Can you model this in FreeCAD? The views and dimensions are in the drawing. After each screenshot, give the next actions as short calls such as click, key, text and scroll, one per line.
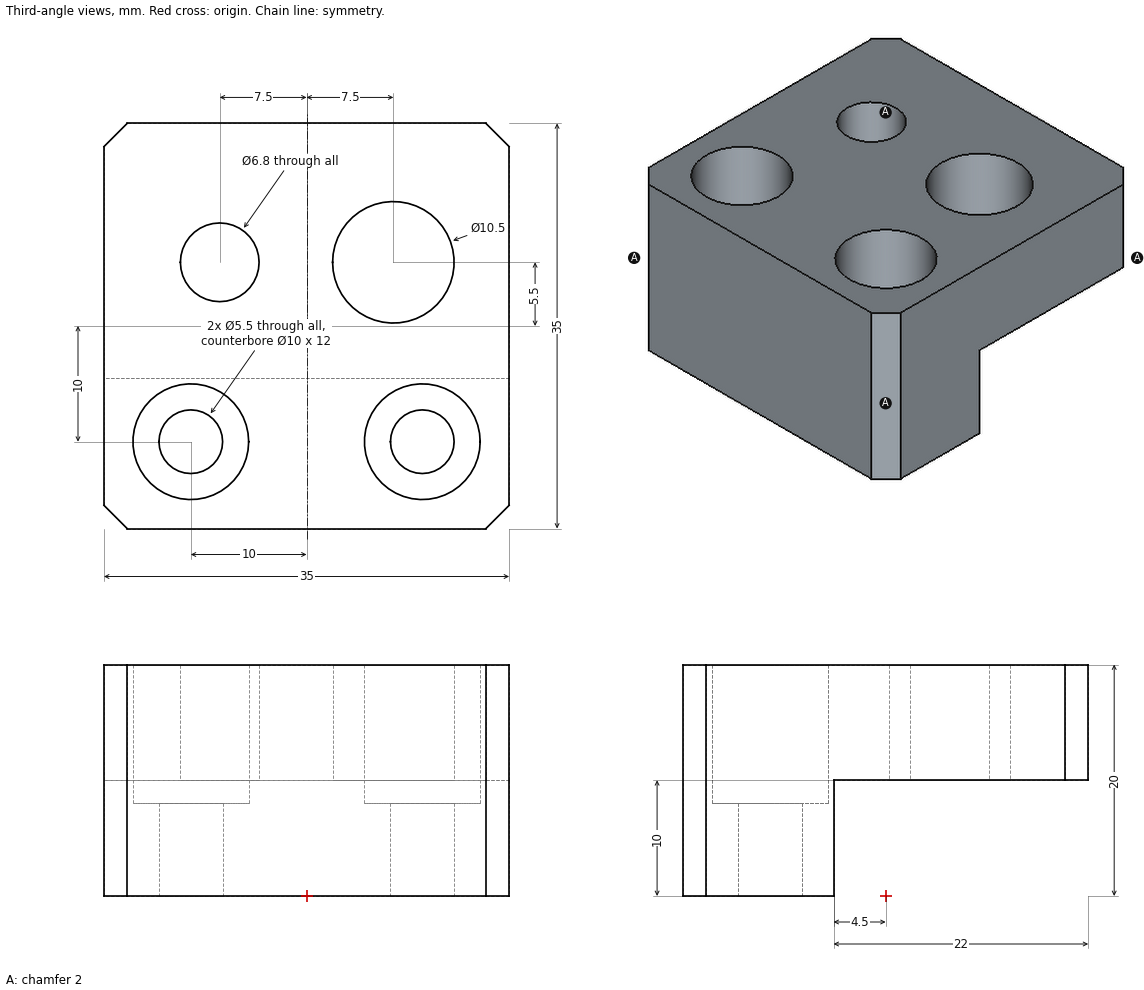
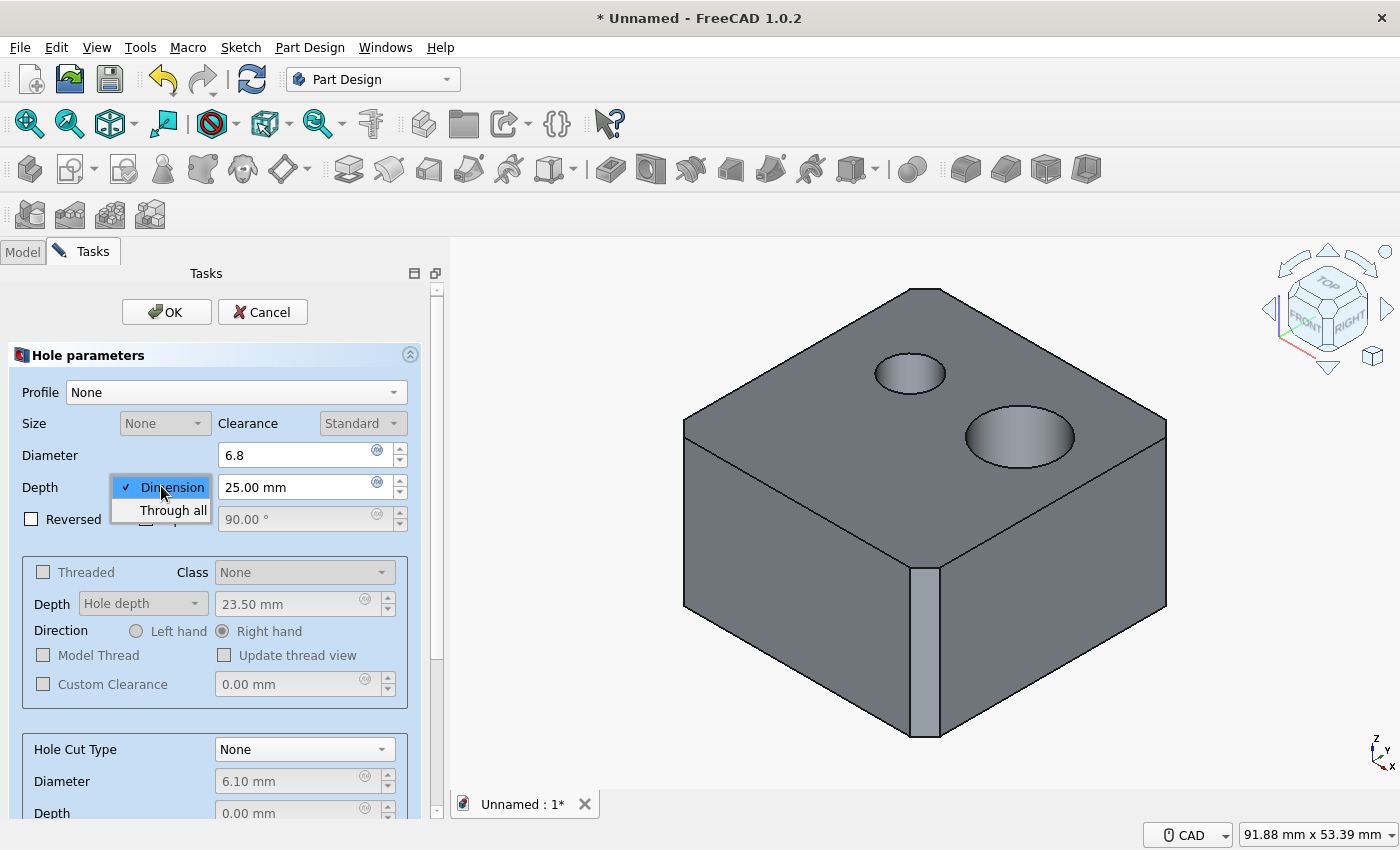
click(160, 510)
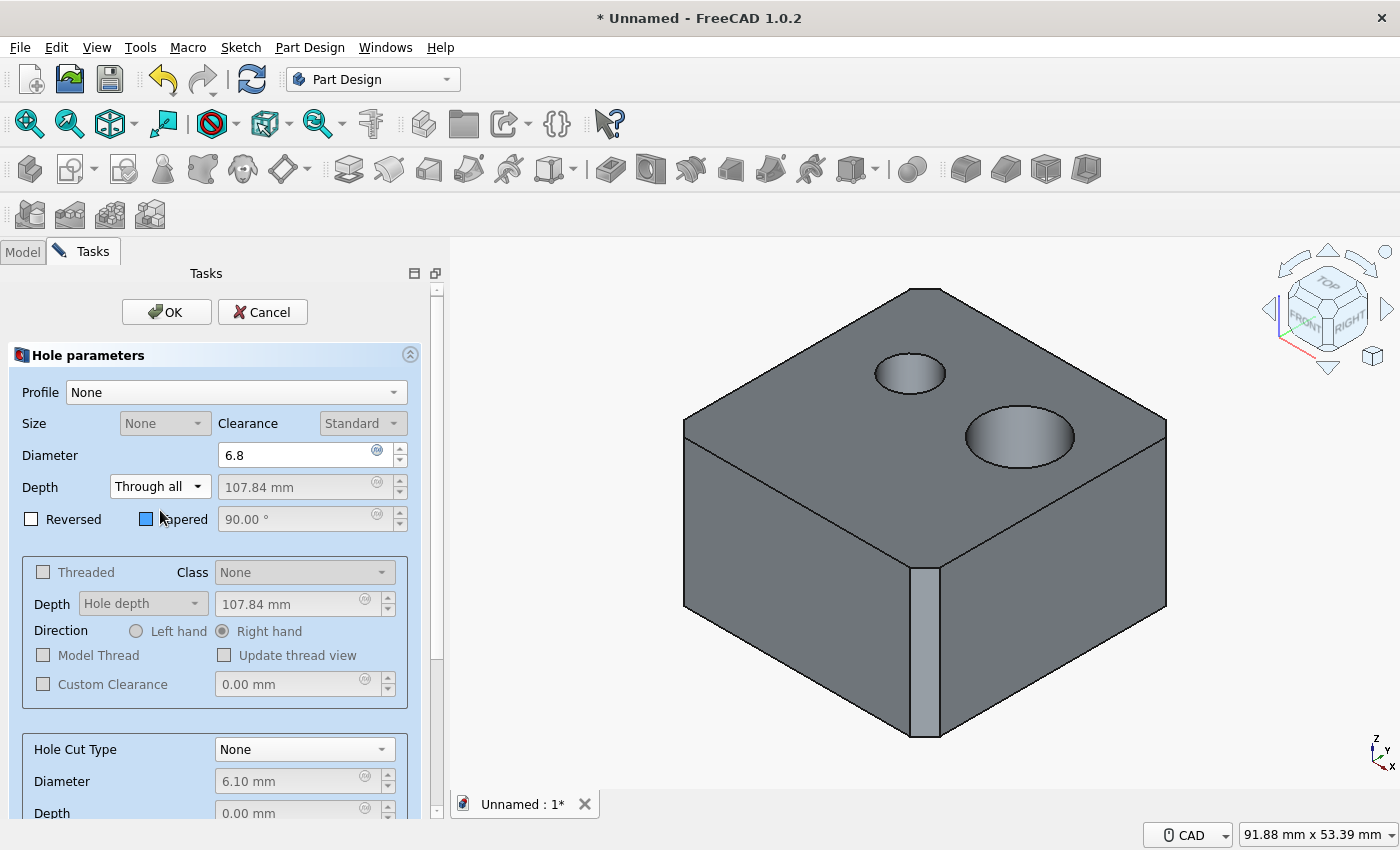
click(167, 312)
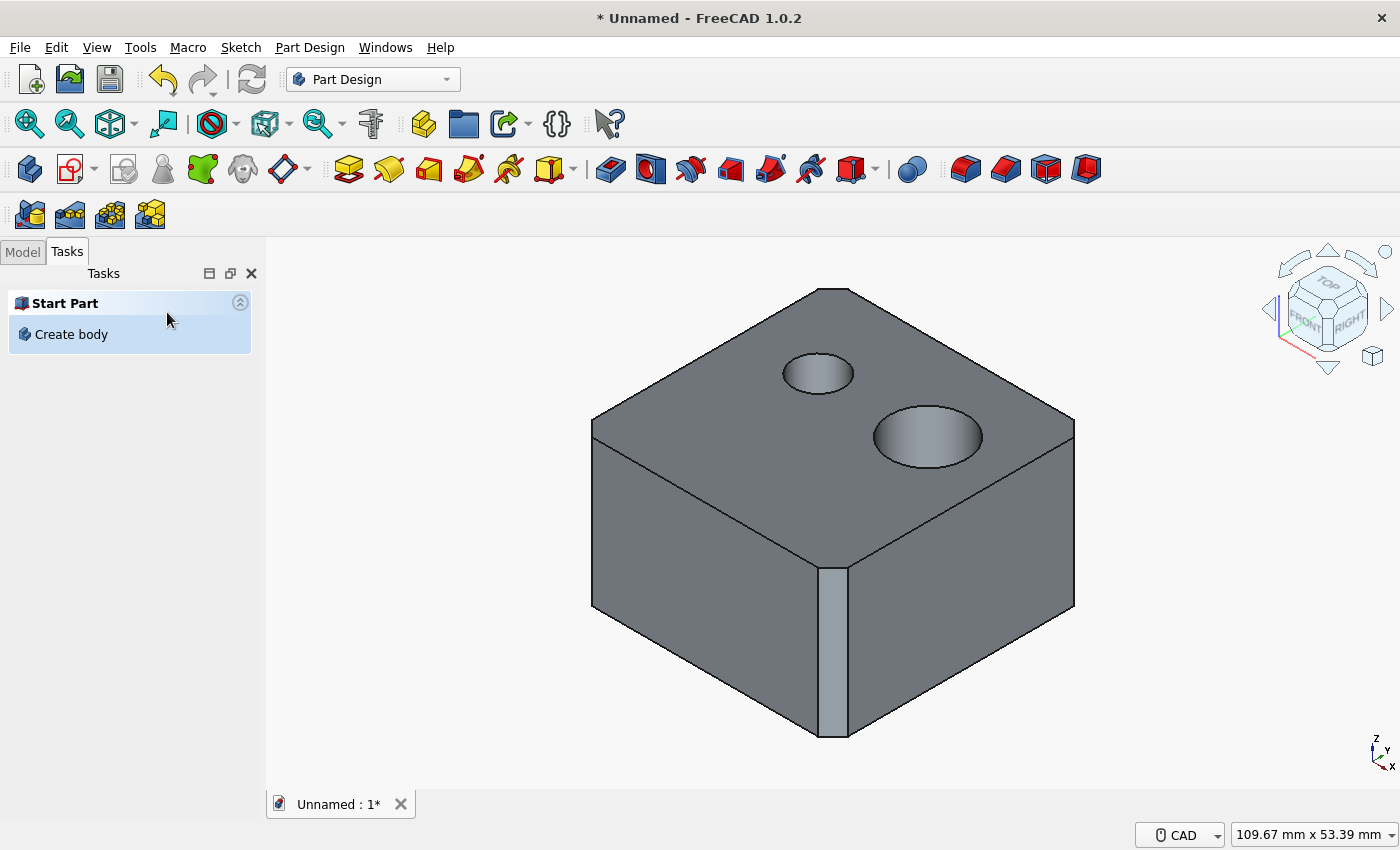
click(796, 449)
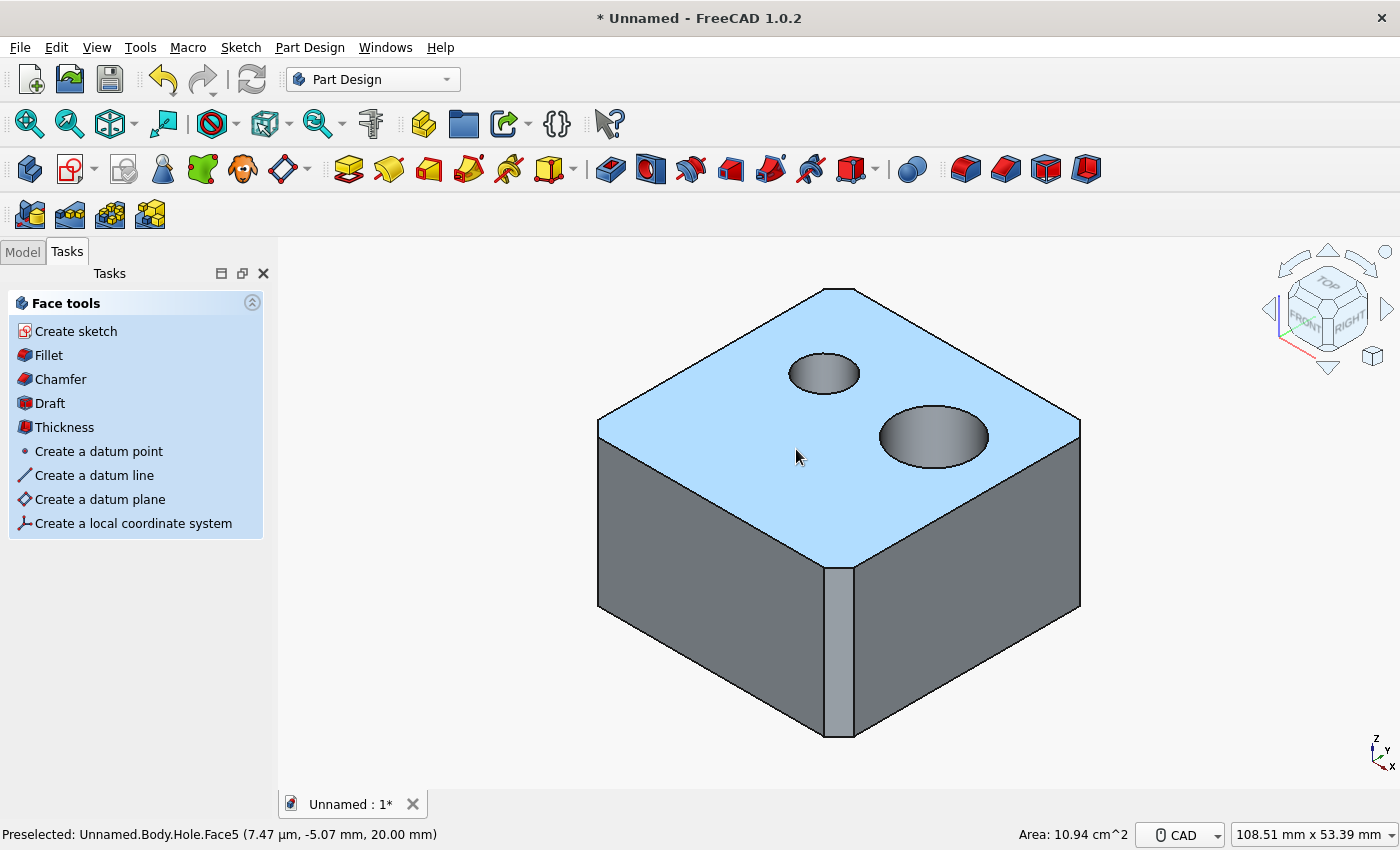
click(70, 170)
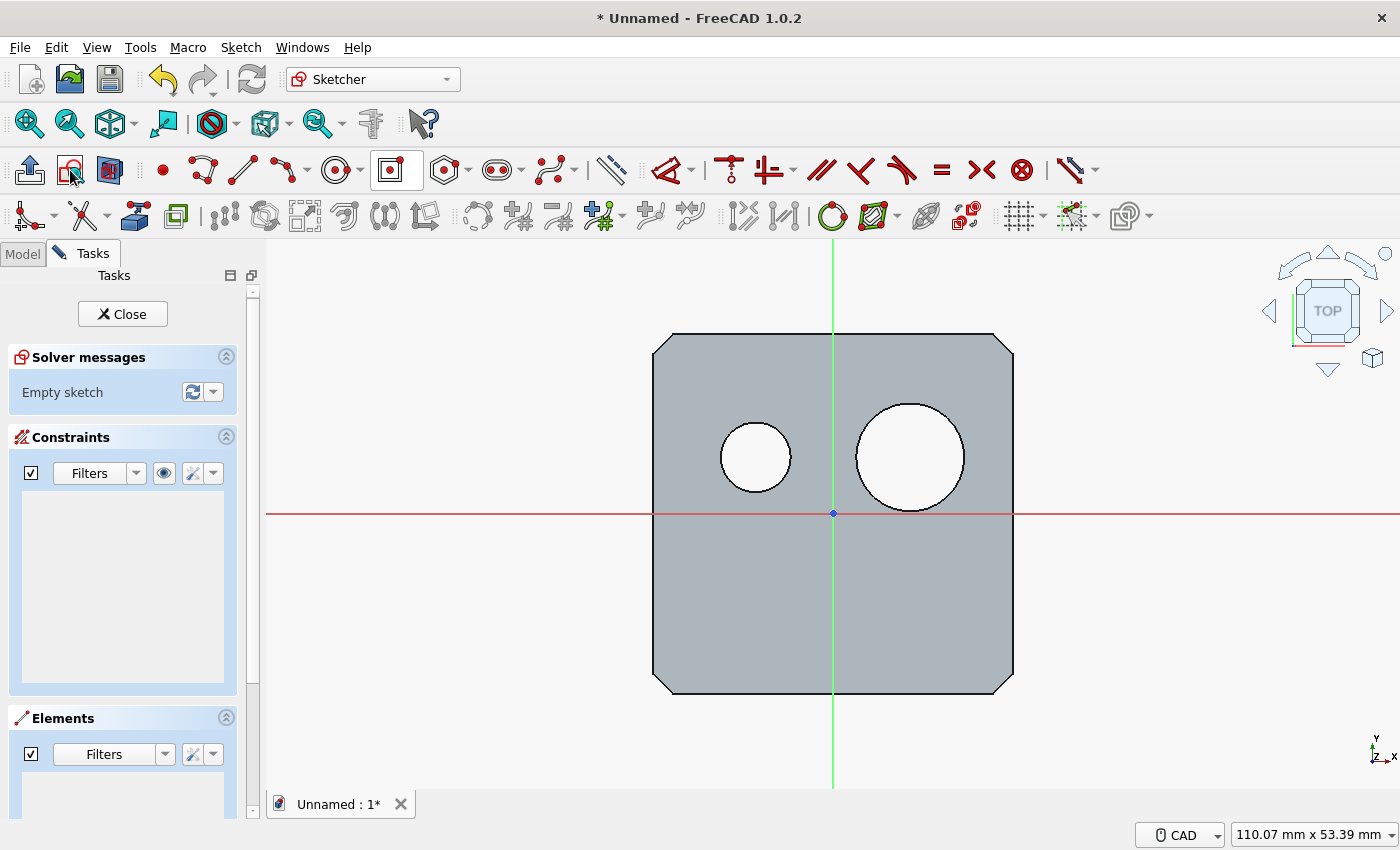
scroll(873, 618, up, 5)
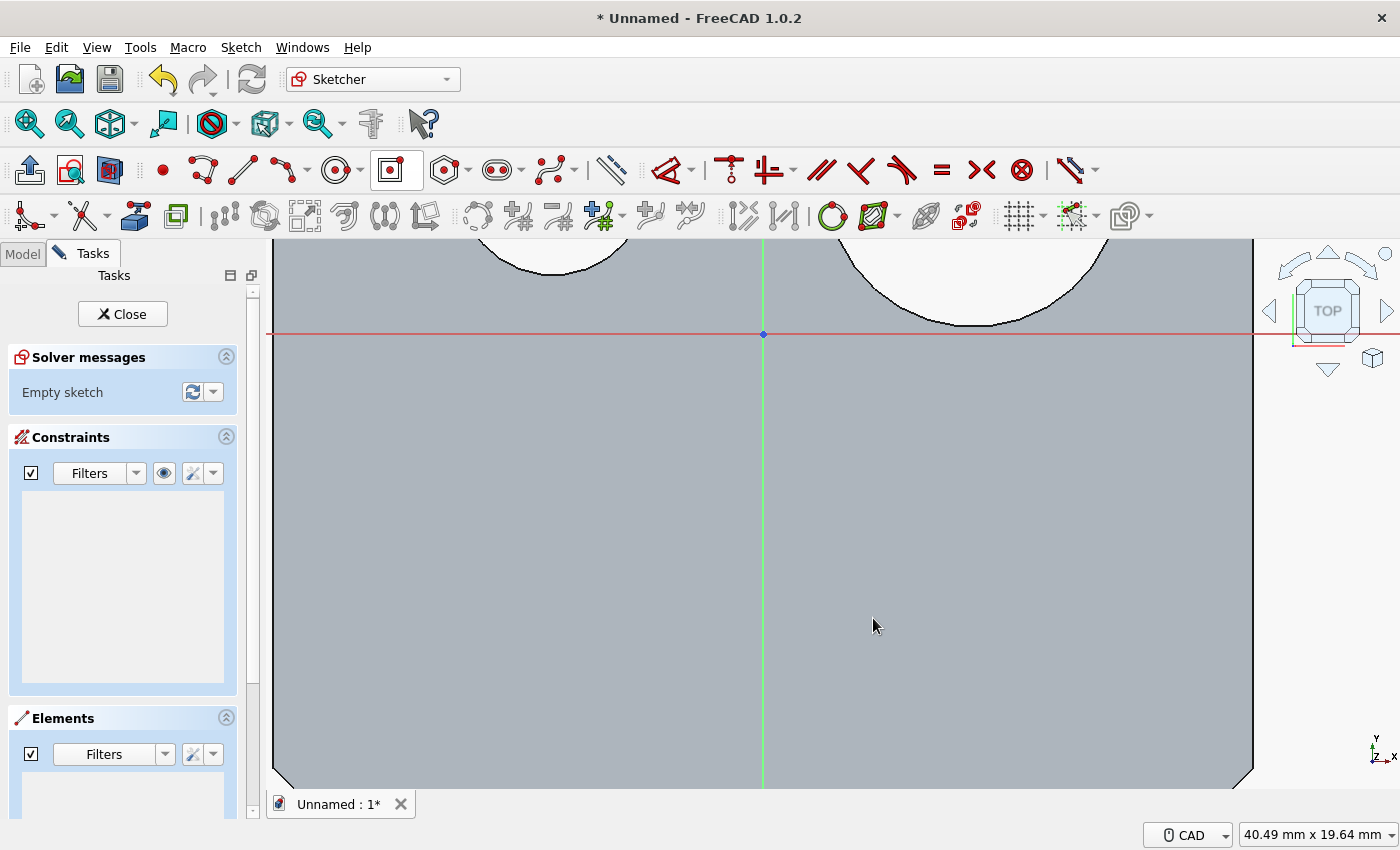
key(g)
key(c)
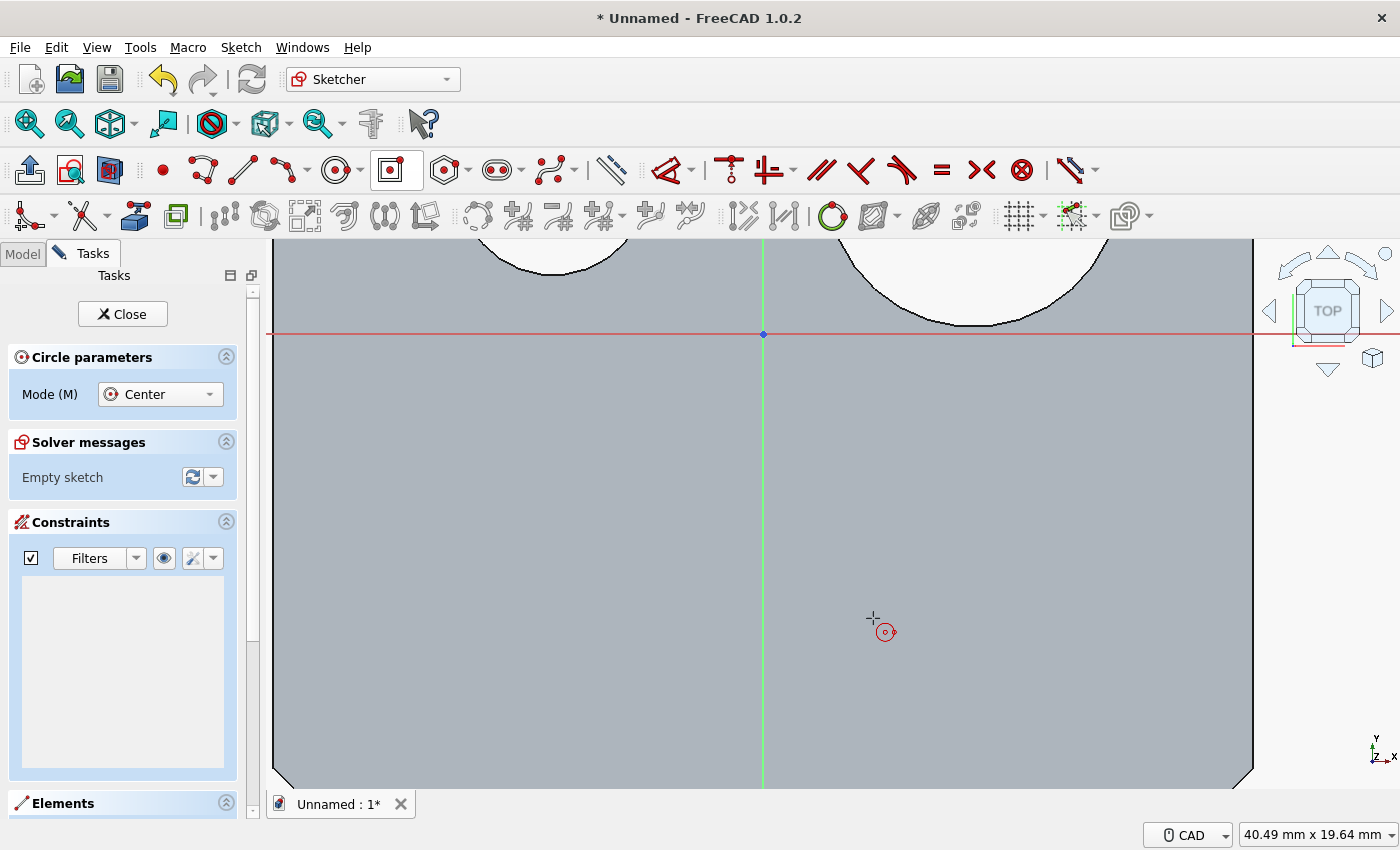
click(483, 614)
move(538, 560)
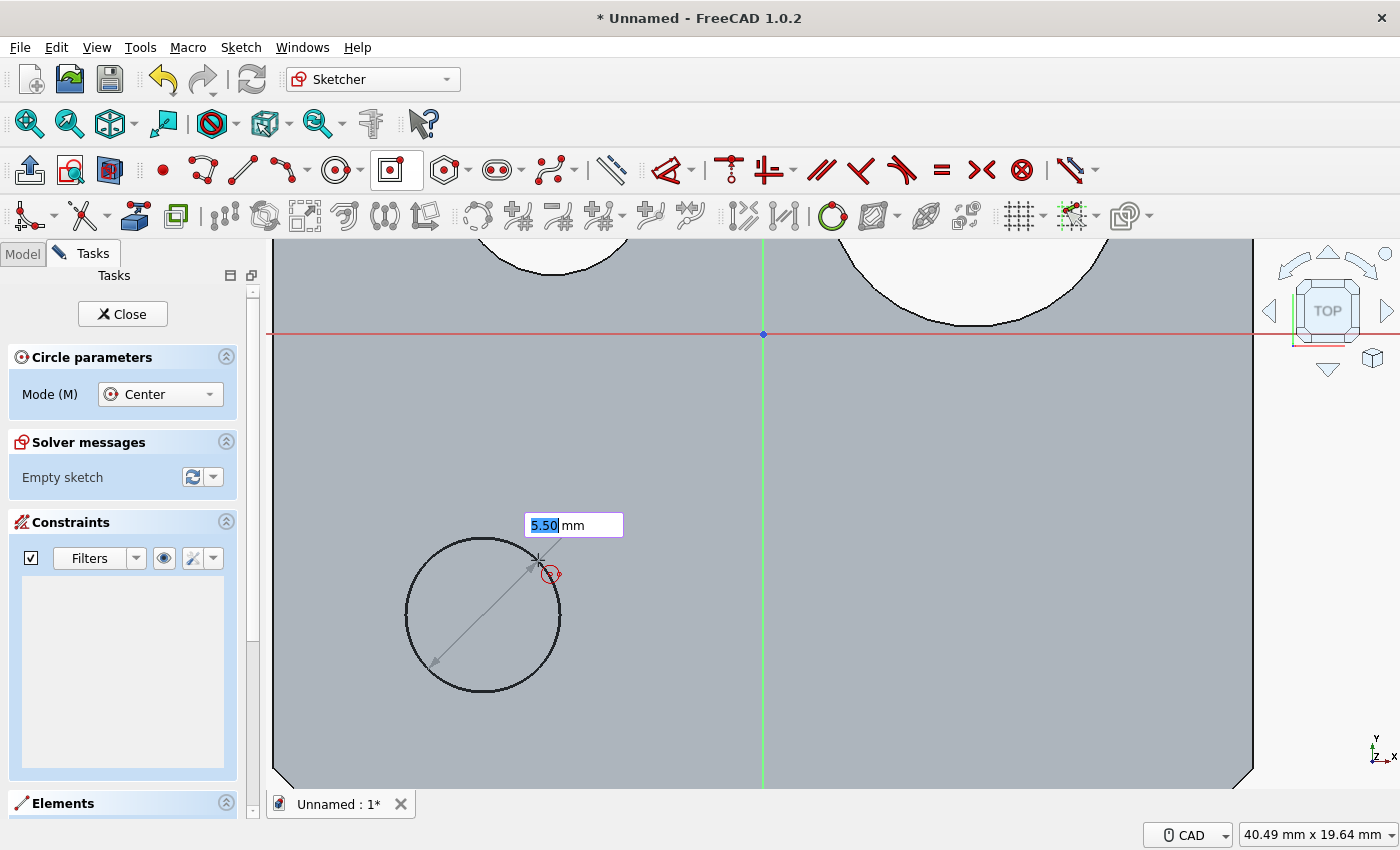
text(5.5)
key(Return)